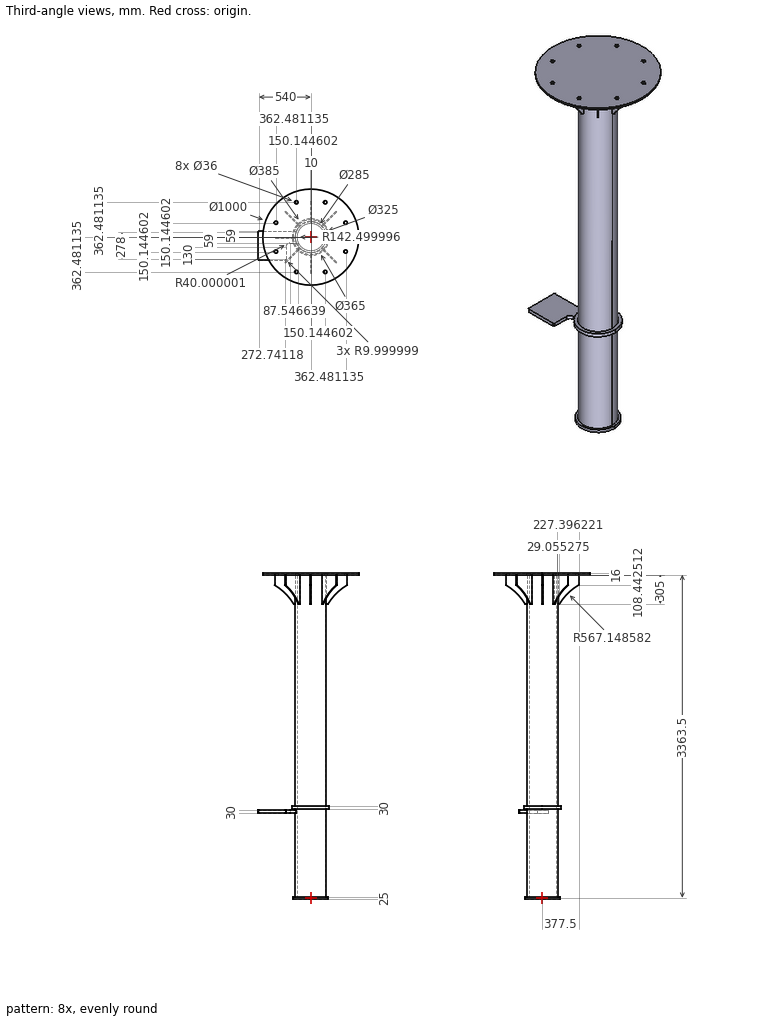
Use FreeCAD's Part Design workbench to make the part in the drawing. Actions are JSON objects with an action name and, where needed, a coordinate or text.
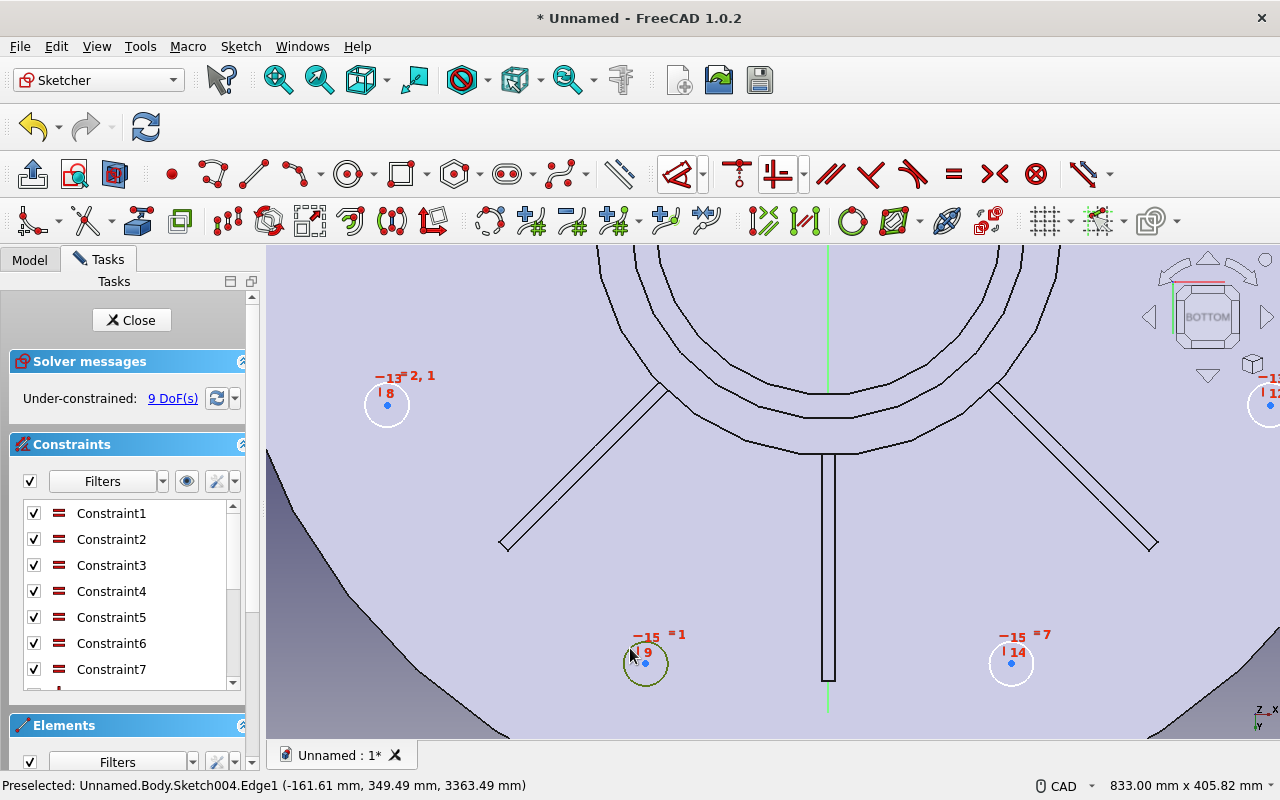
{"action": "key", "text": "k o"}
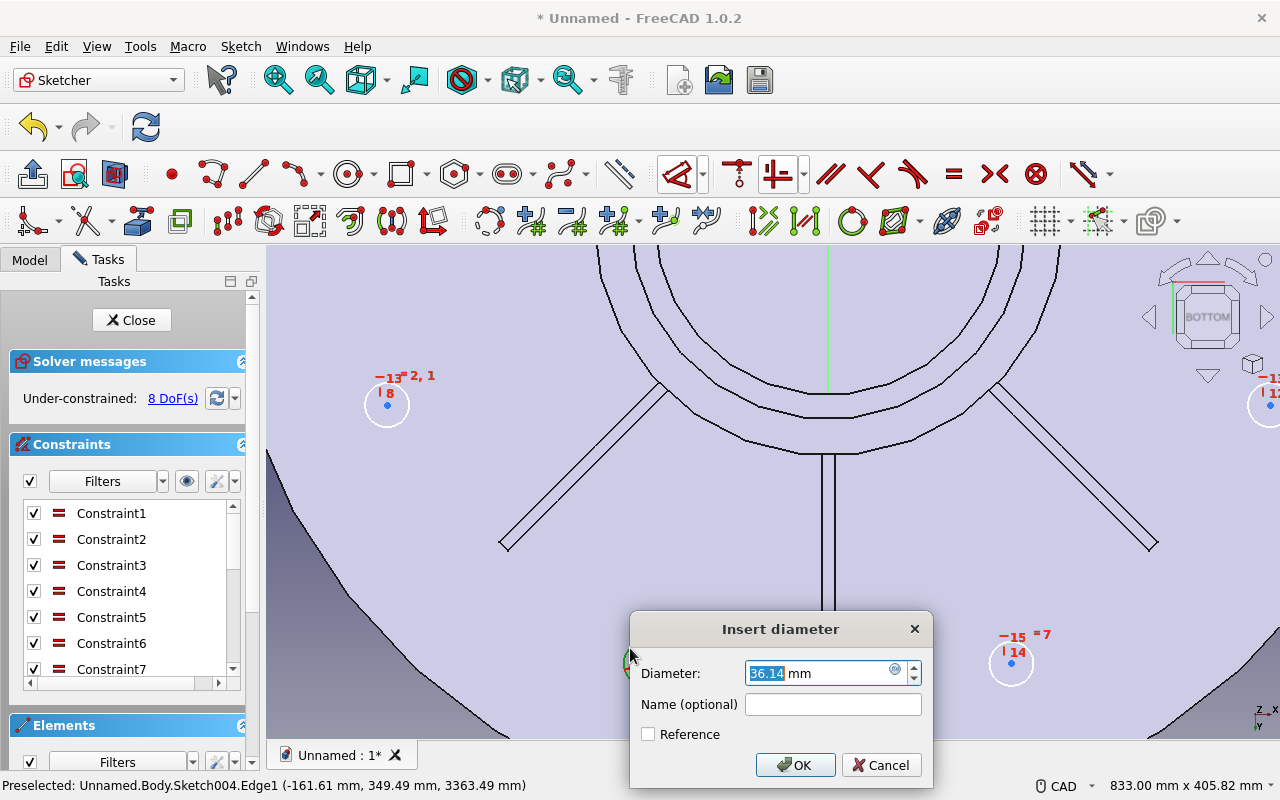
{"action": "type", "text": "36"}
{"action": "key", "text": "Return"}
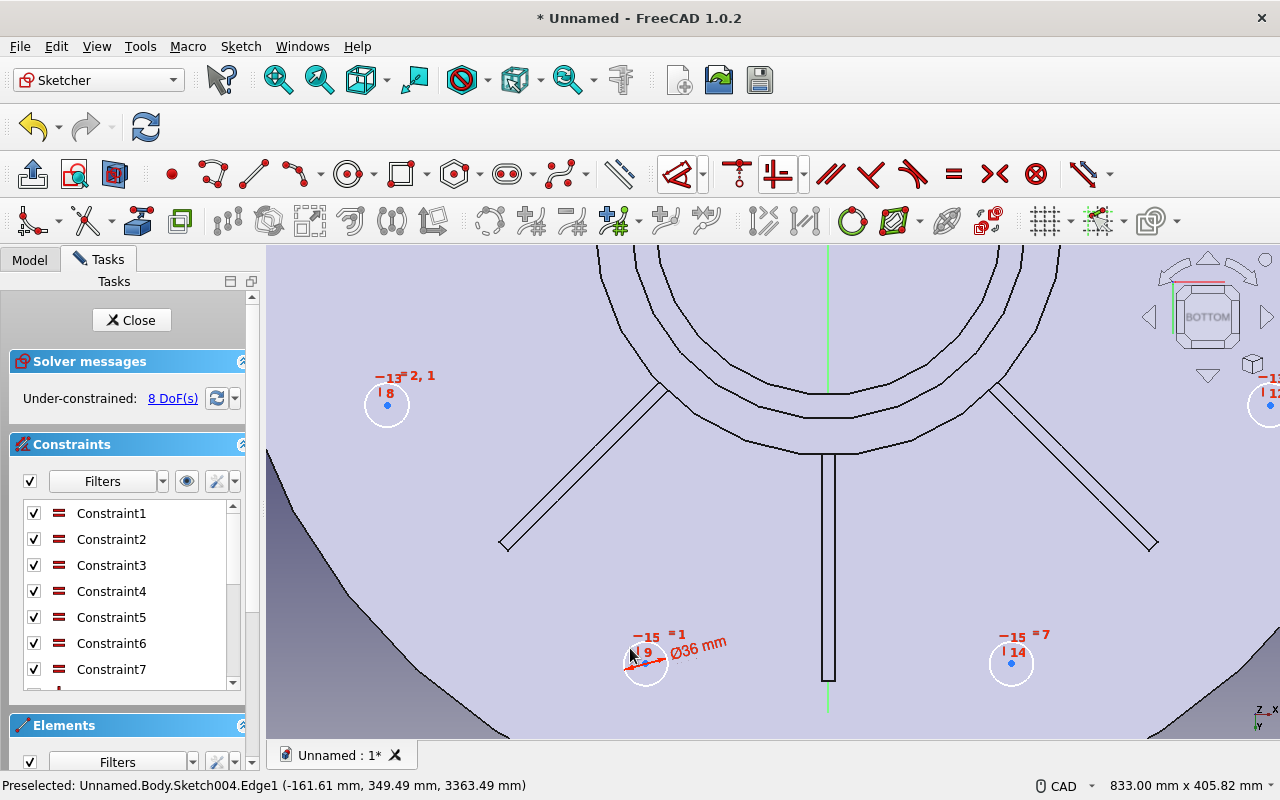
{"action": "left_click", "coordinate": [646, 664]}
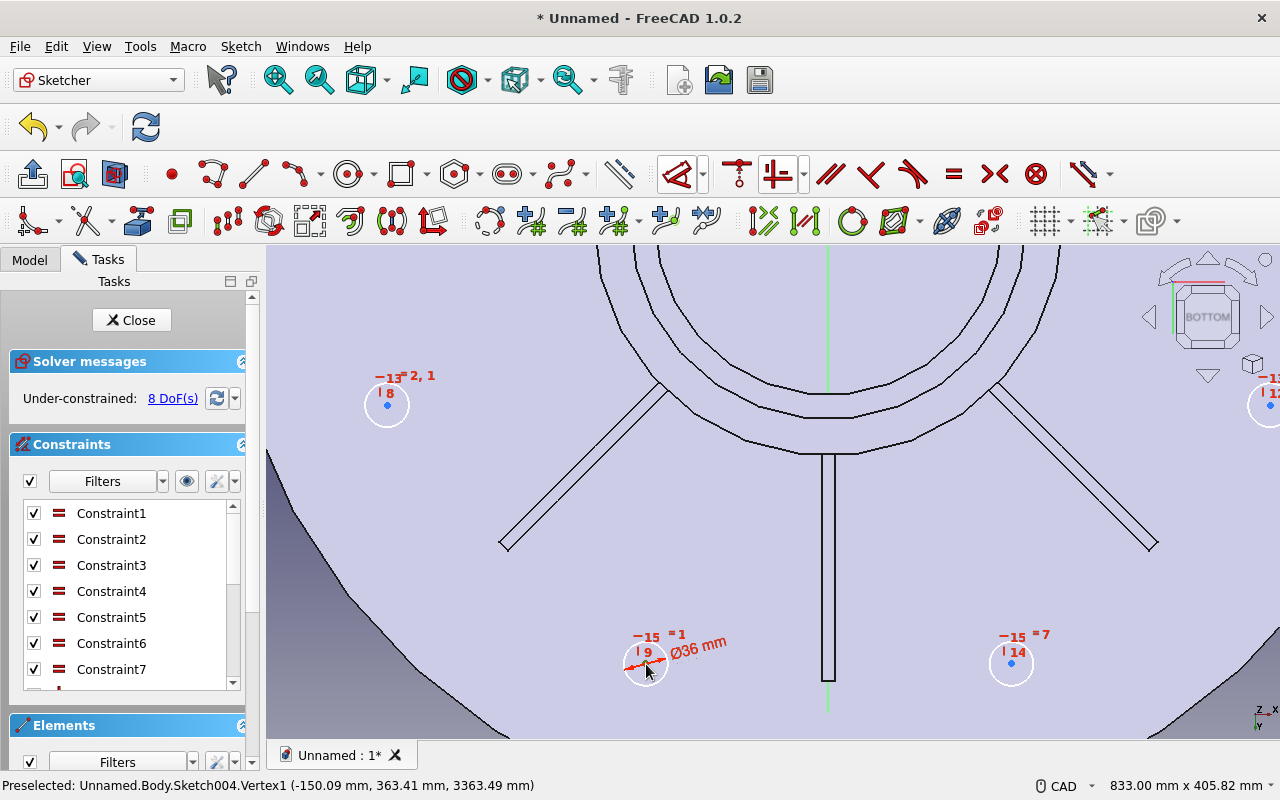
{"action": "key", "text": "l"}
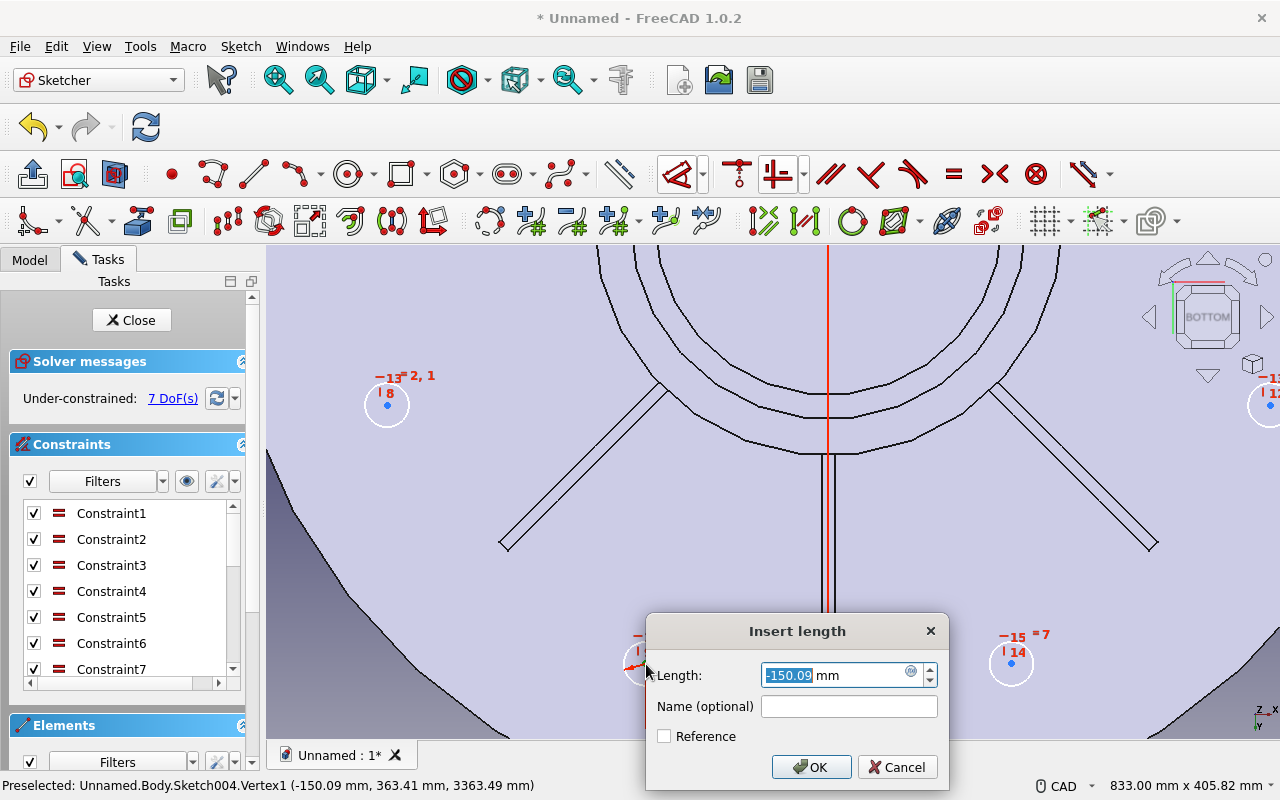
{"action": "type", "text": "-150.144602"}
{"action": "key", "text": "Return"}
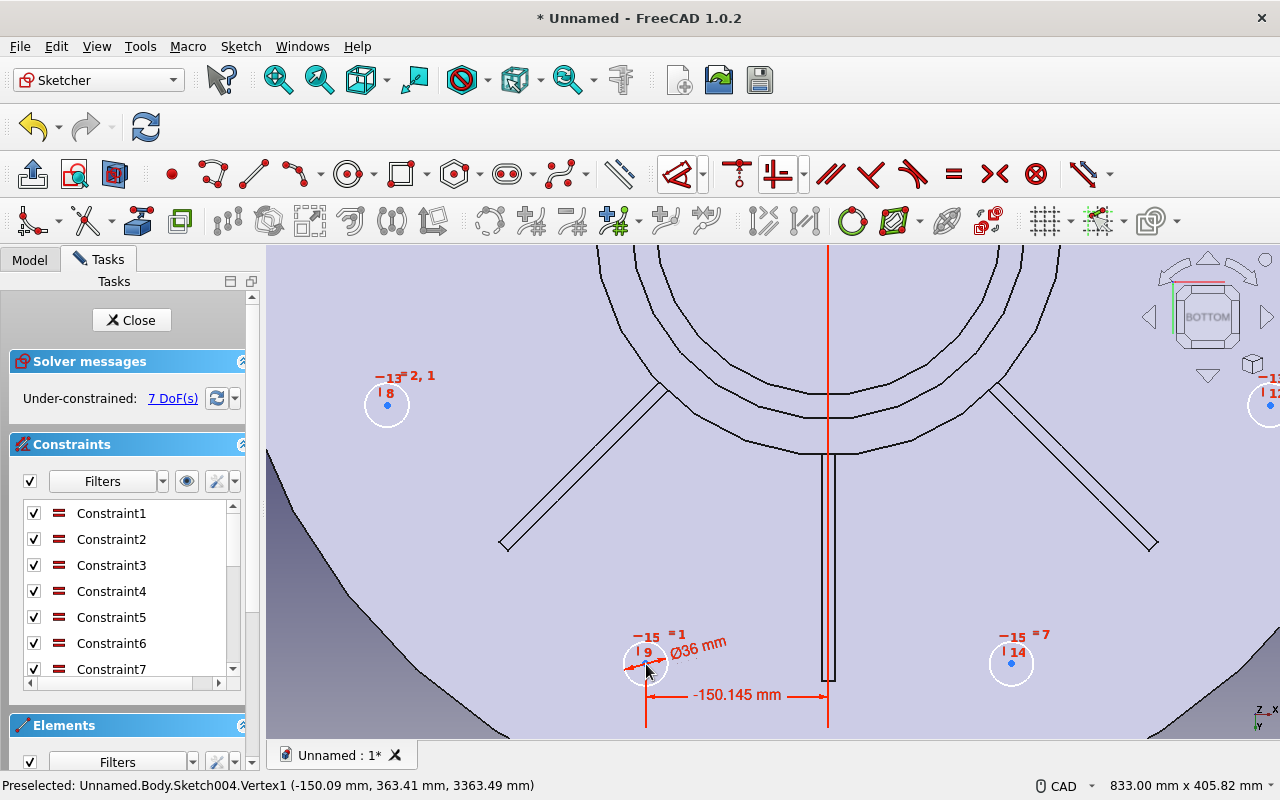
{"action": "left_click", "coordinate": [646, 664]}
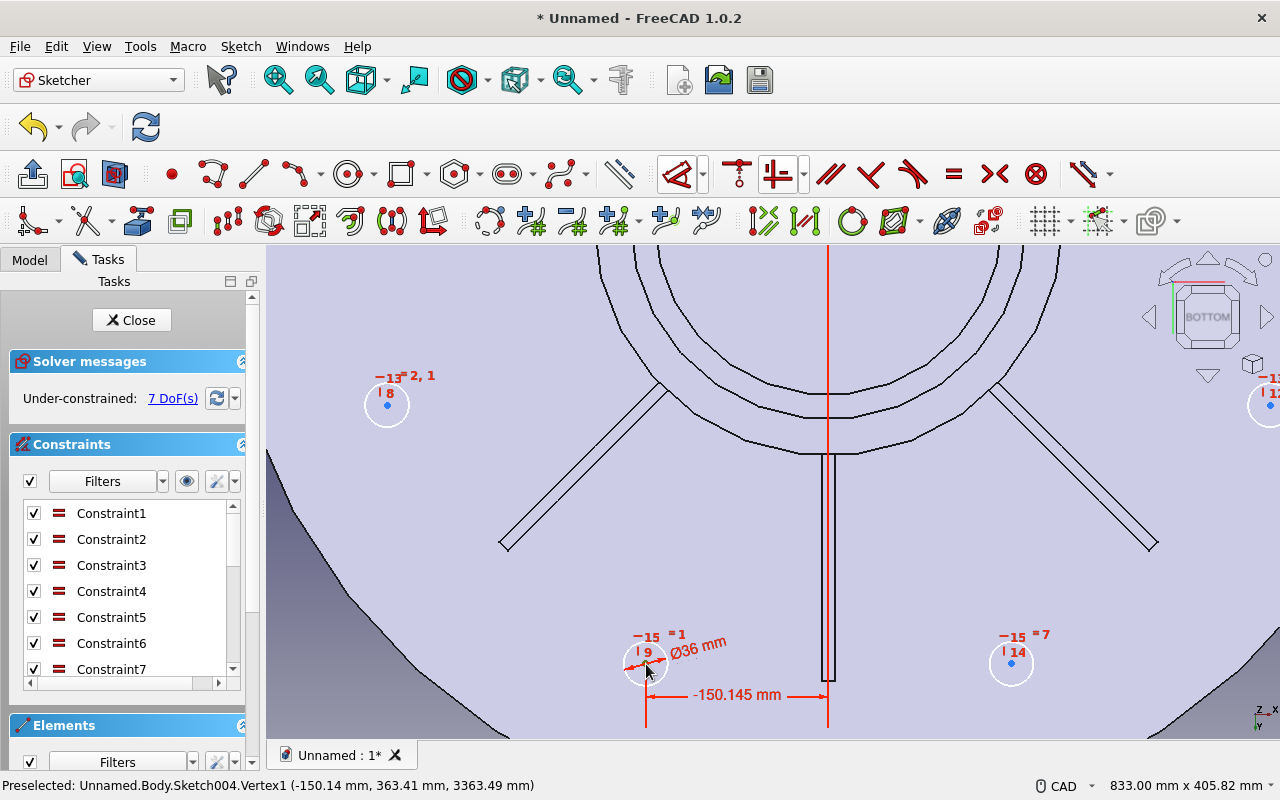
{"action": "key", "text": "i"}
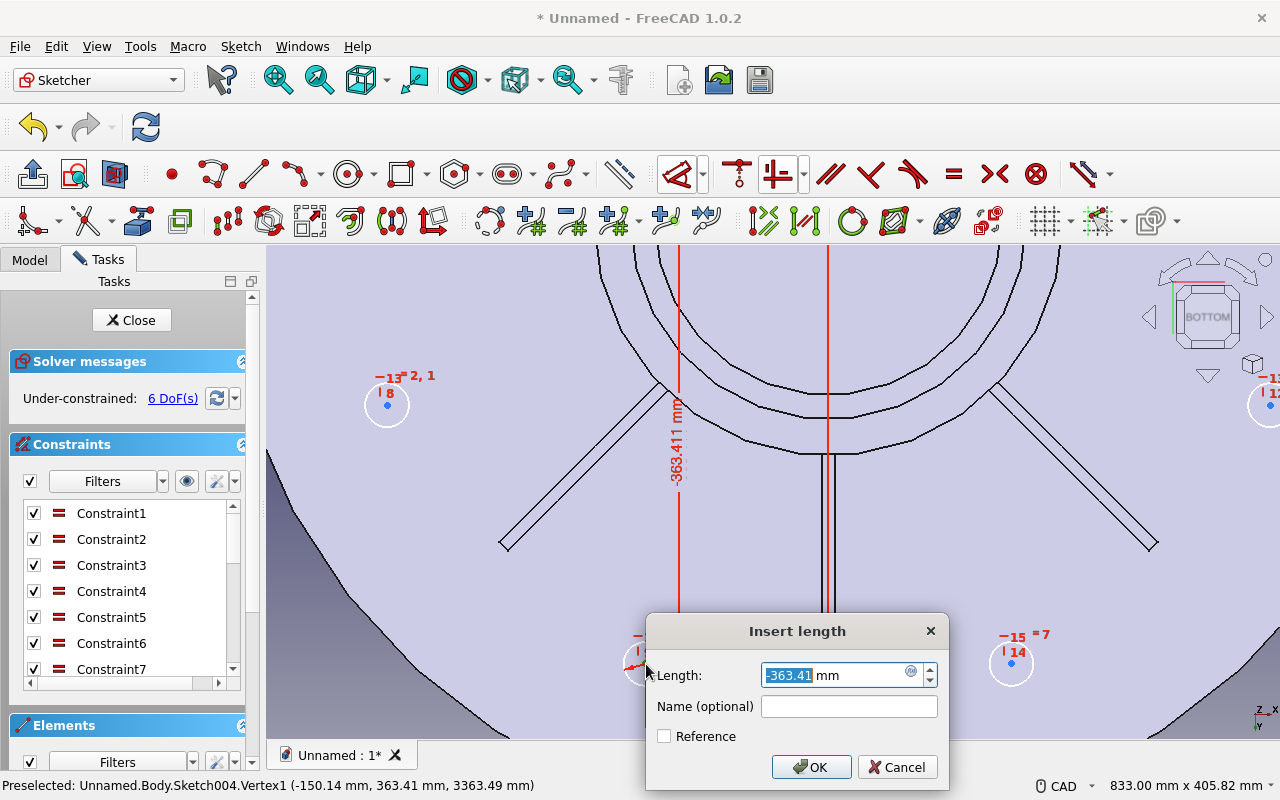
{"action": "type", "text": "-362.481135"}
{"action": "key", "text": "Return"}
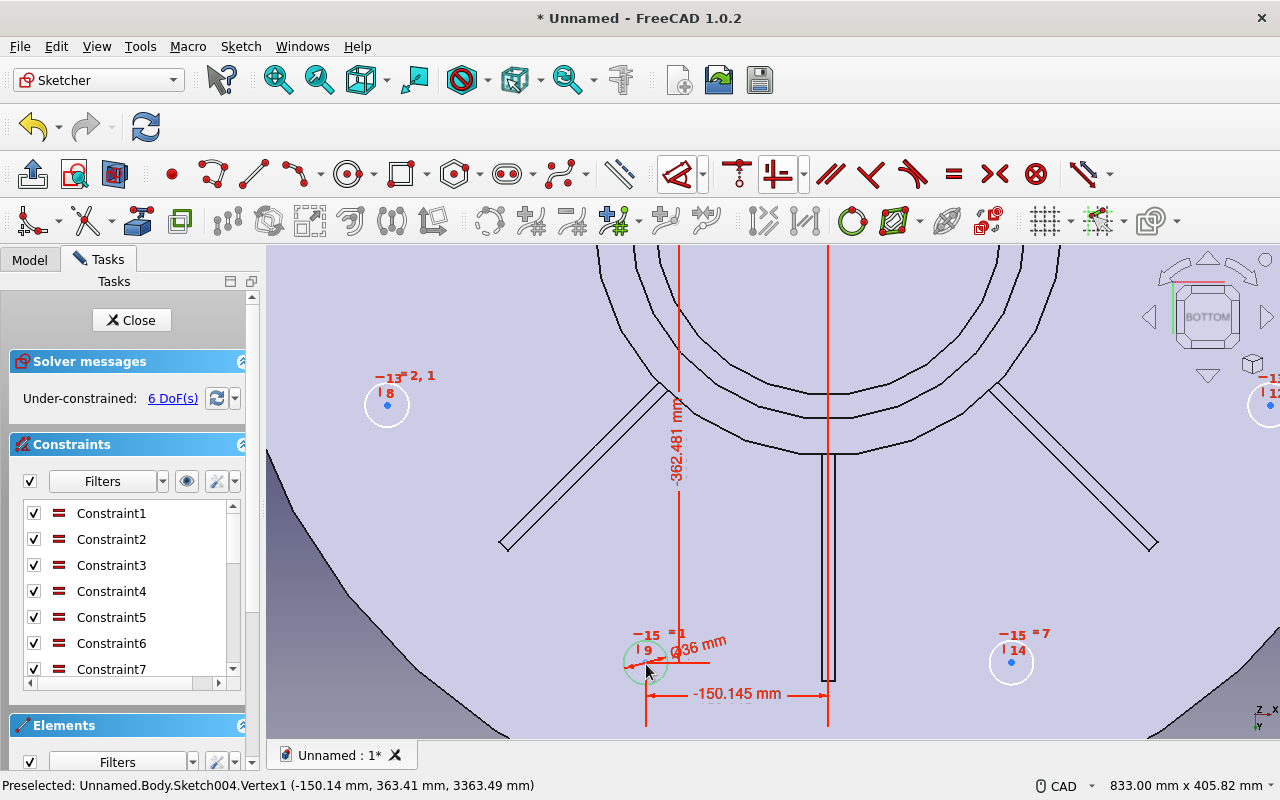
{"action": "left_click", "coordinate": [387, 405]}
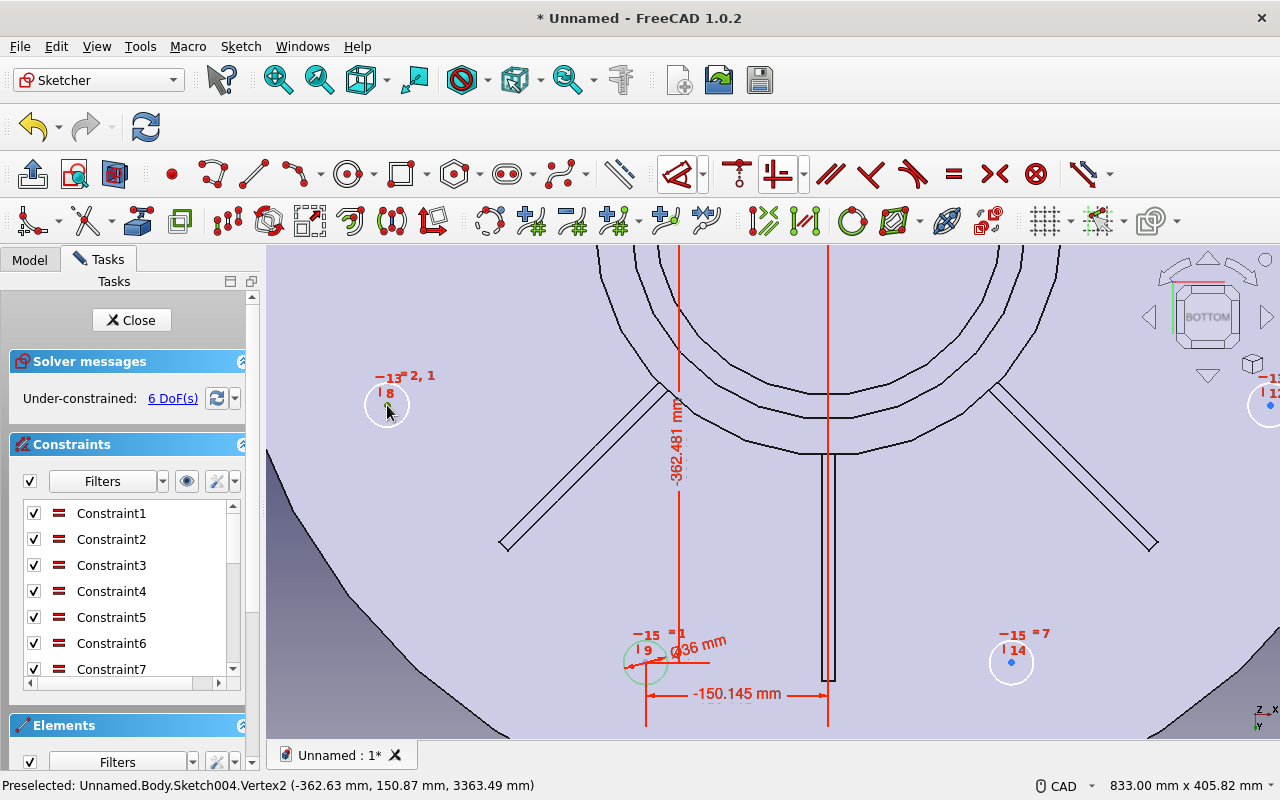
{"action": "key", "text": "l"}